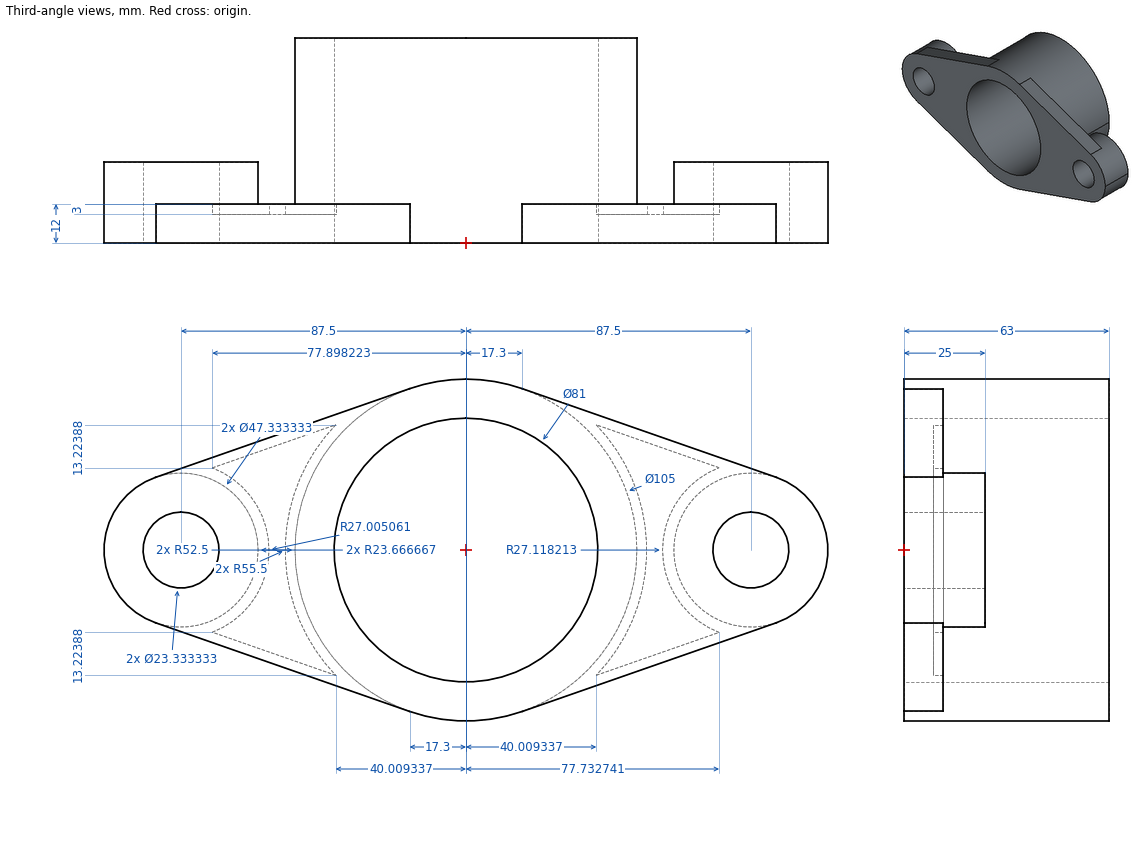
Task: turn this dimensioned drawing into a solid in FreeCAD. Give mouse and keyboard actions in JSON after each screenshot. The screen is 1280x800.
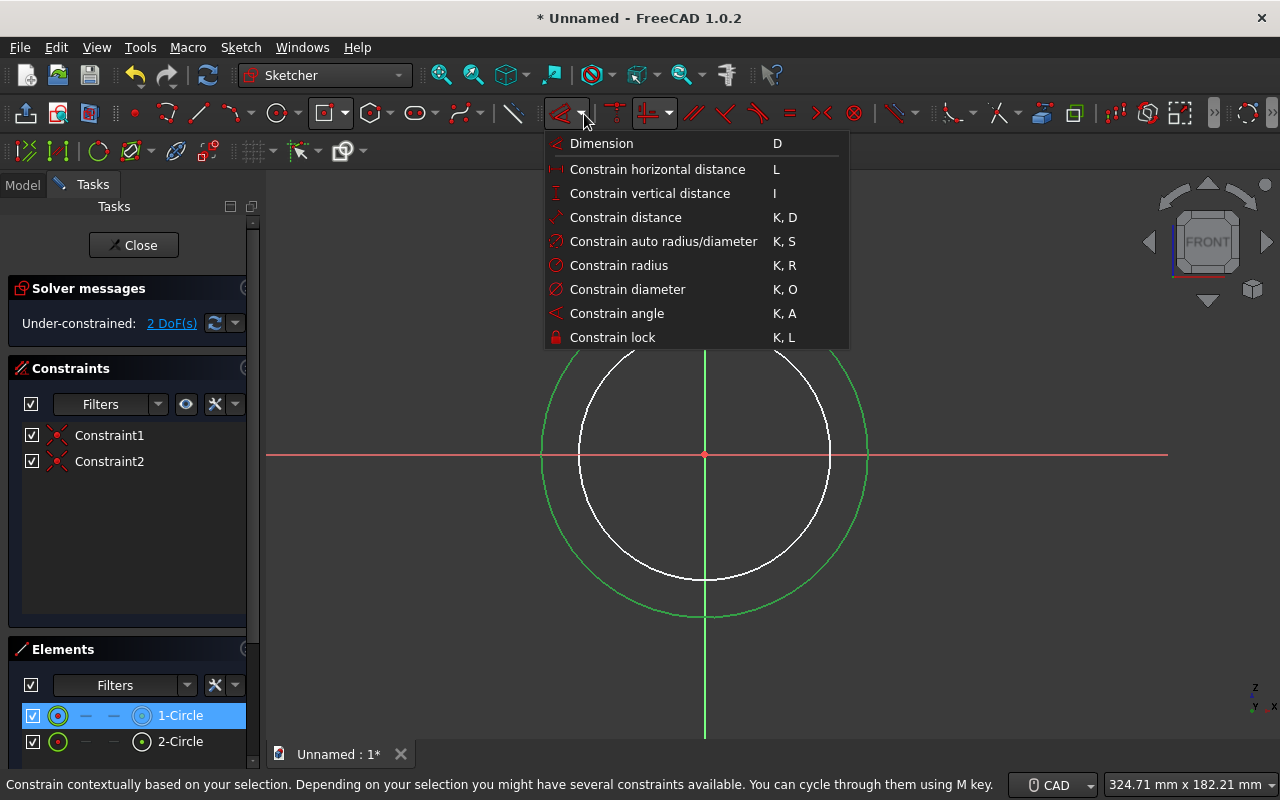
{"action": "left_click", "coordinate": [697, 289]}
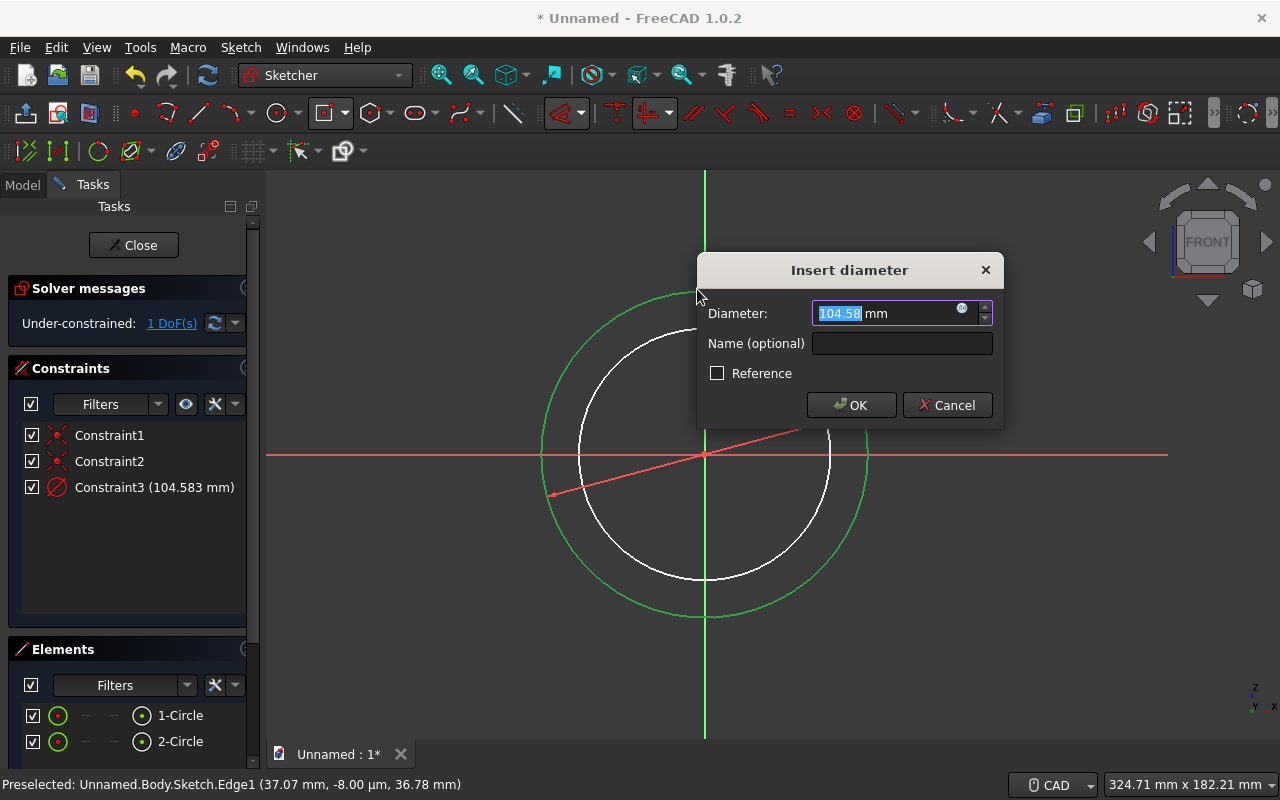
{"action": "type", "text": "105"}
{"action": "key", "text": "Return"}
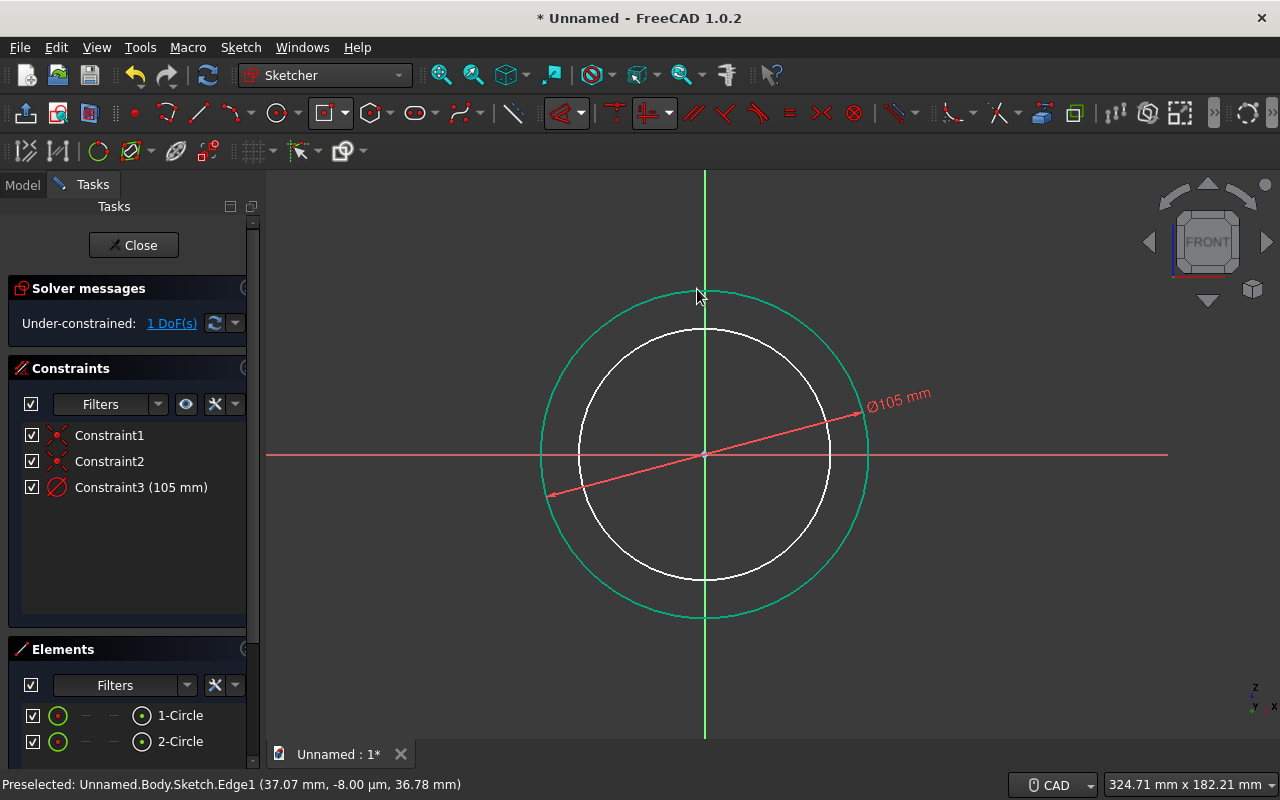
{"action": "left_click", "coordinate": [793, 365]}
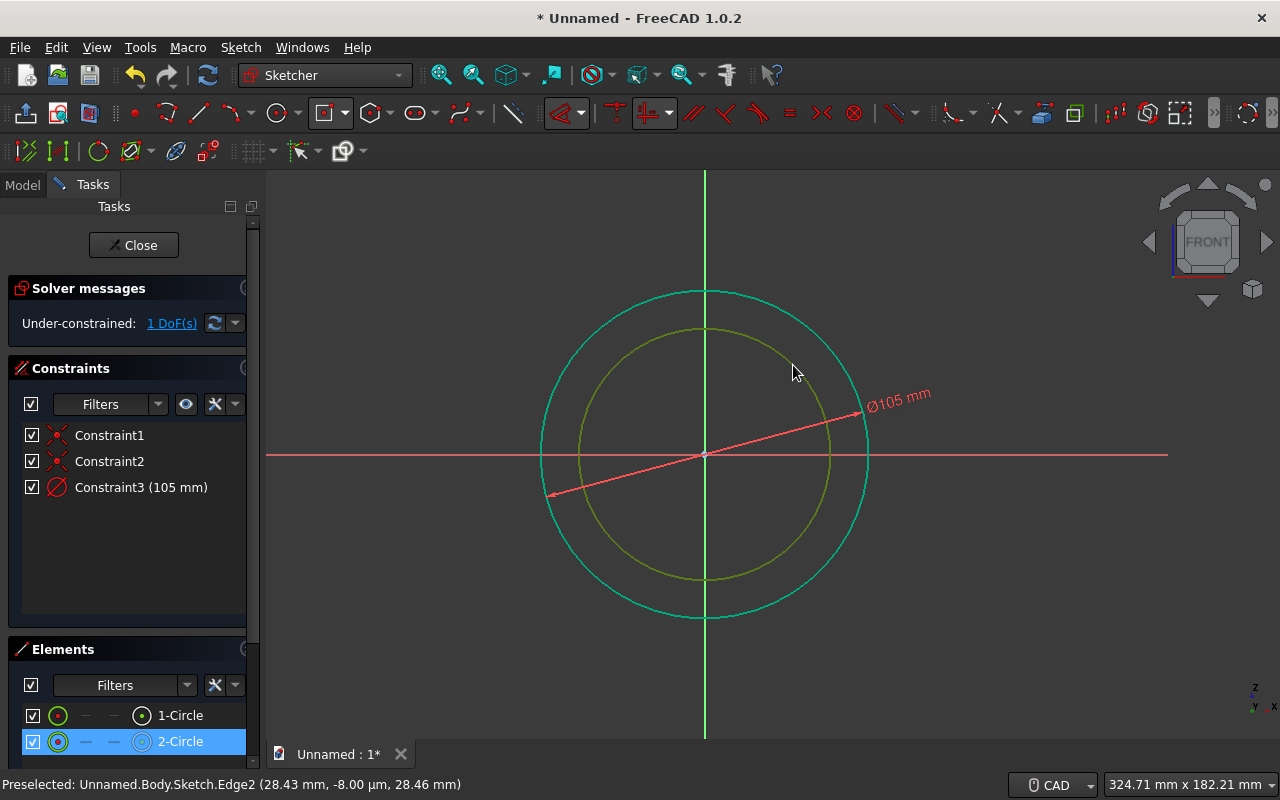
{"action": "key", "text": "k o"}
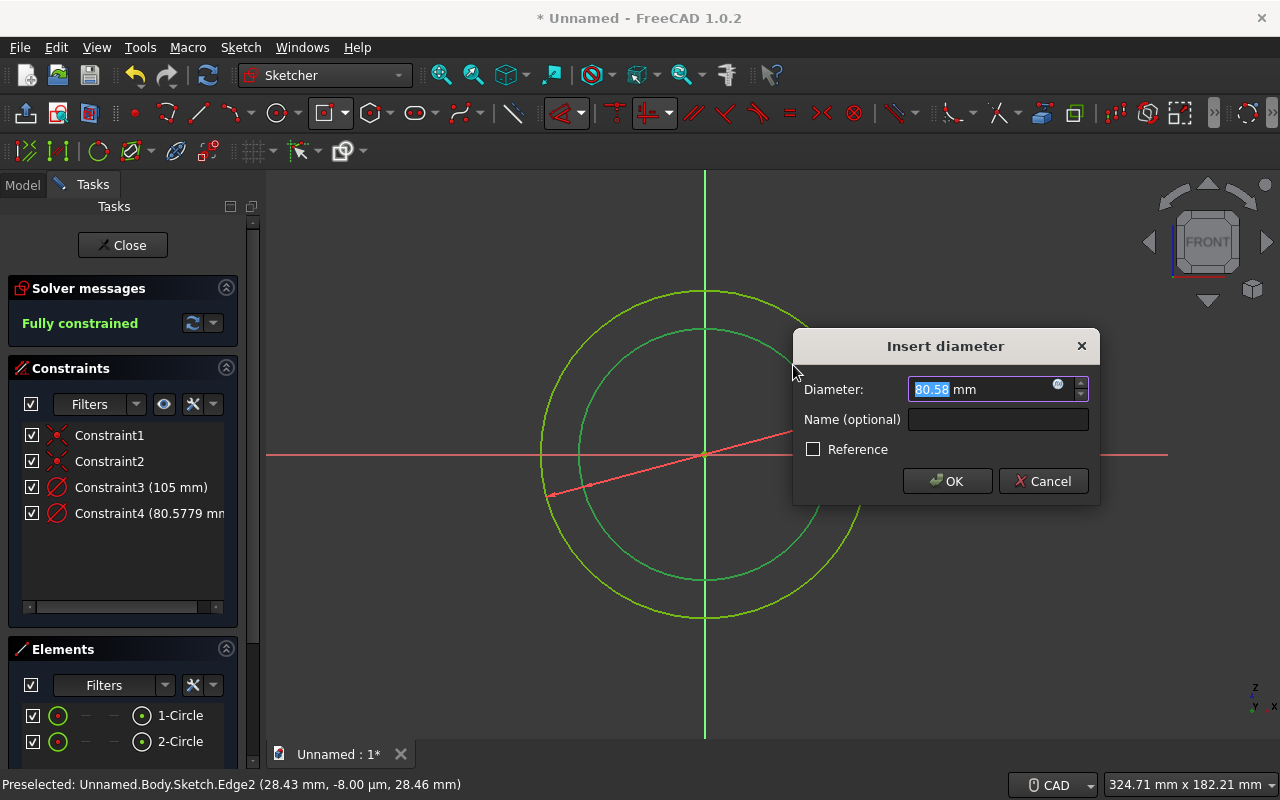
{"action": "type", "text": "81"}
{"action": "key", "text": "Return"}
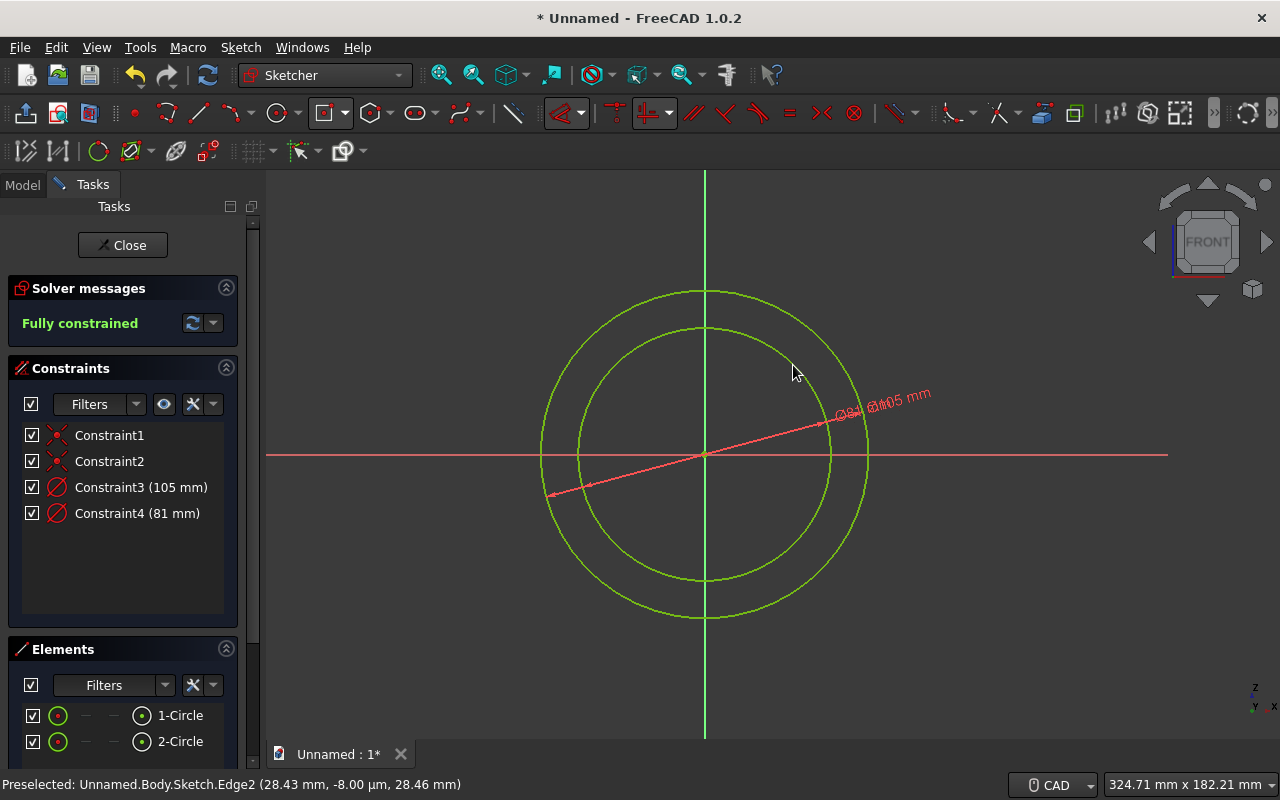
{"action": "left_click", "coordinate": [123, 245]}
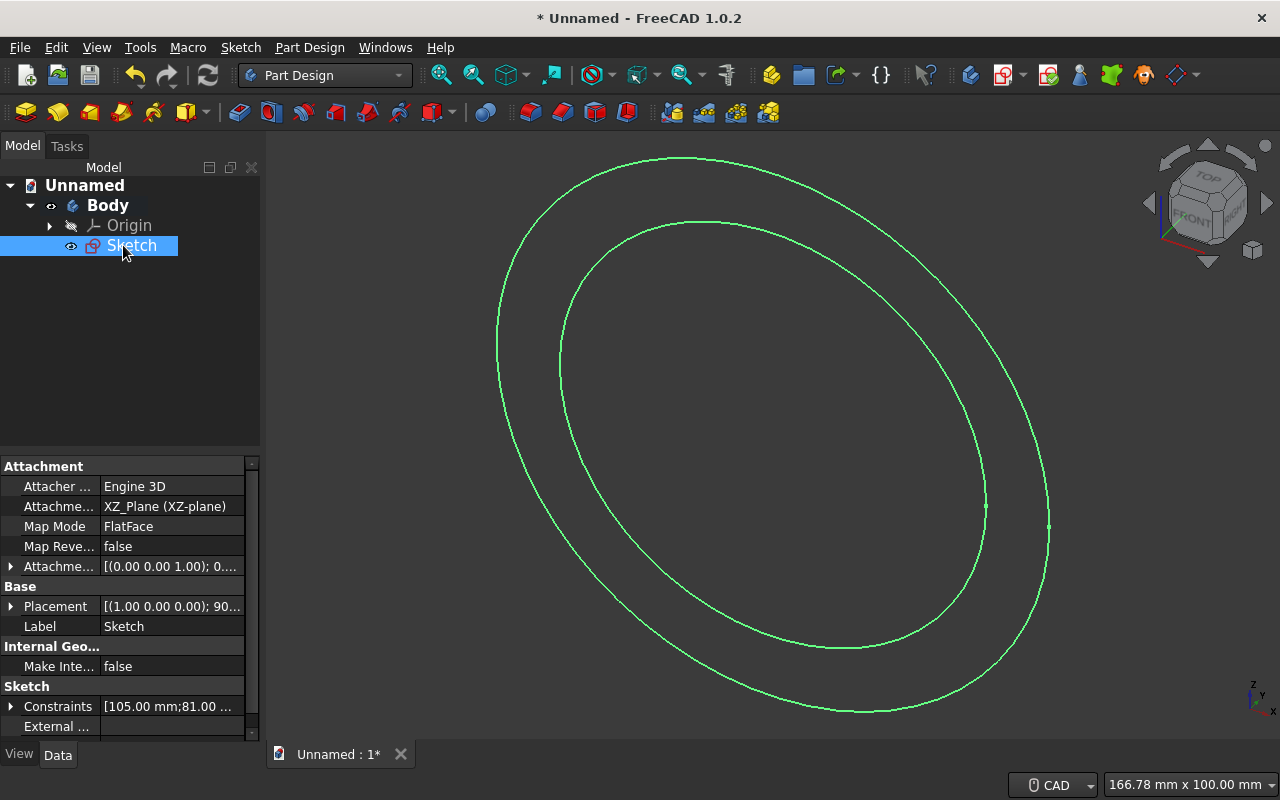
{"action": "left_click", "coordinate": [26, 112]}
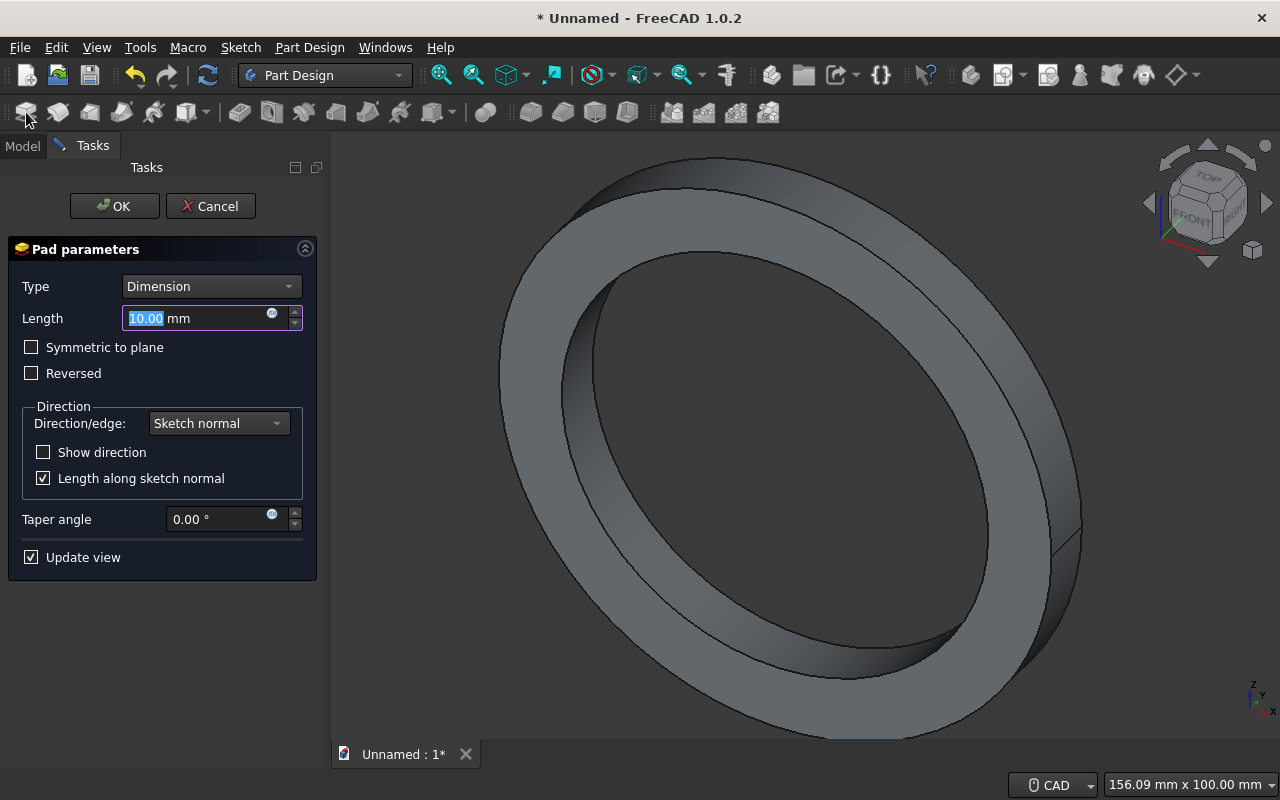
{"action": "type", "text": "63"}
{"action": "key", "text": "Tab"}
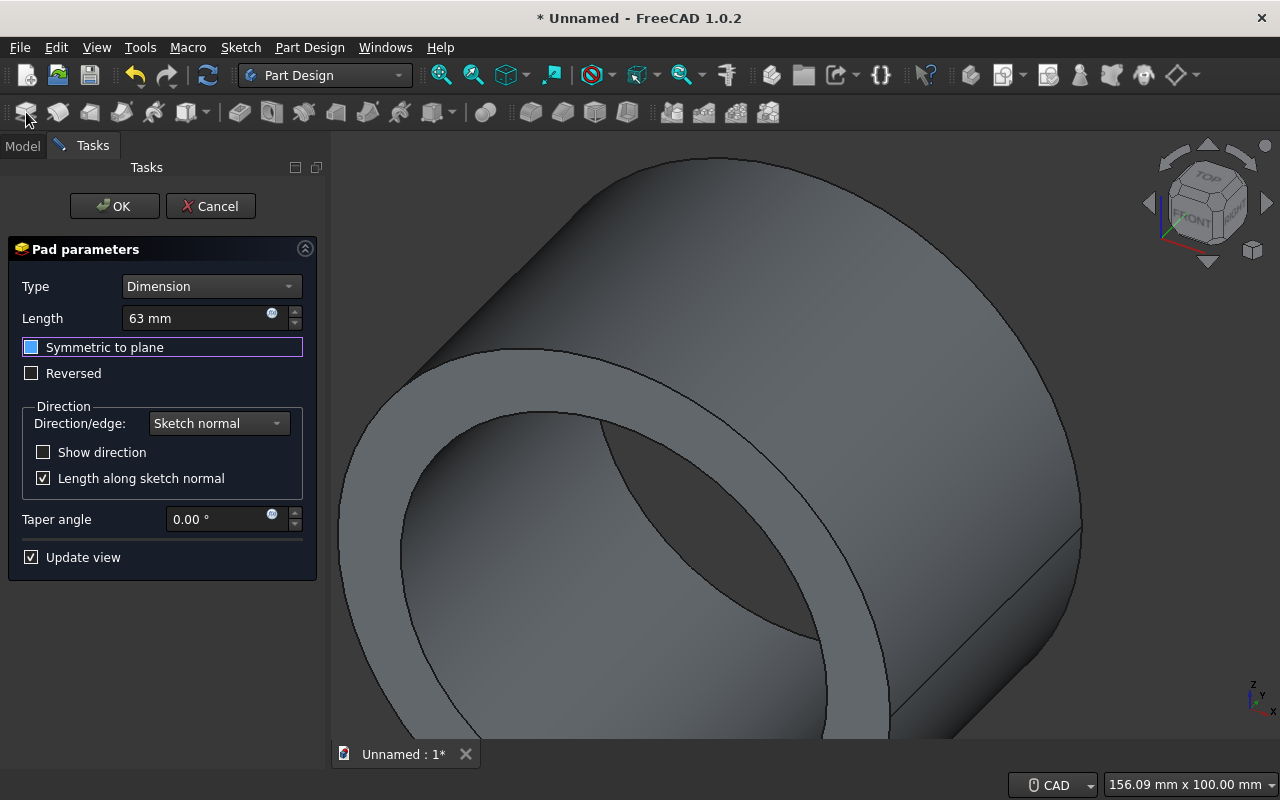
{"action": "left_click", "coordinate": [30, 373]}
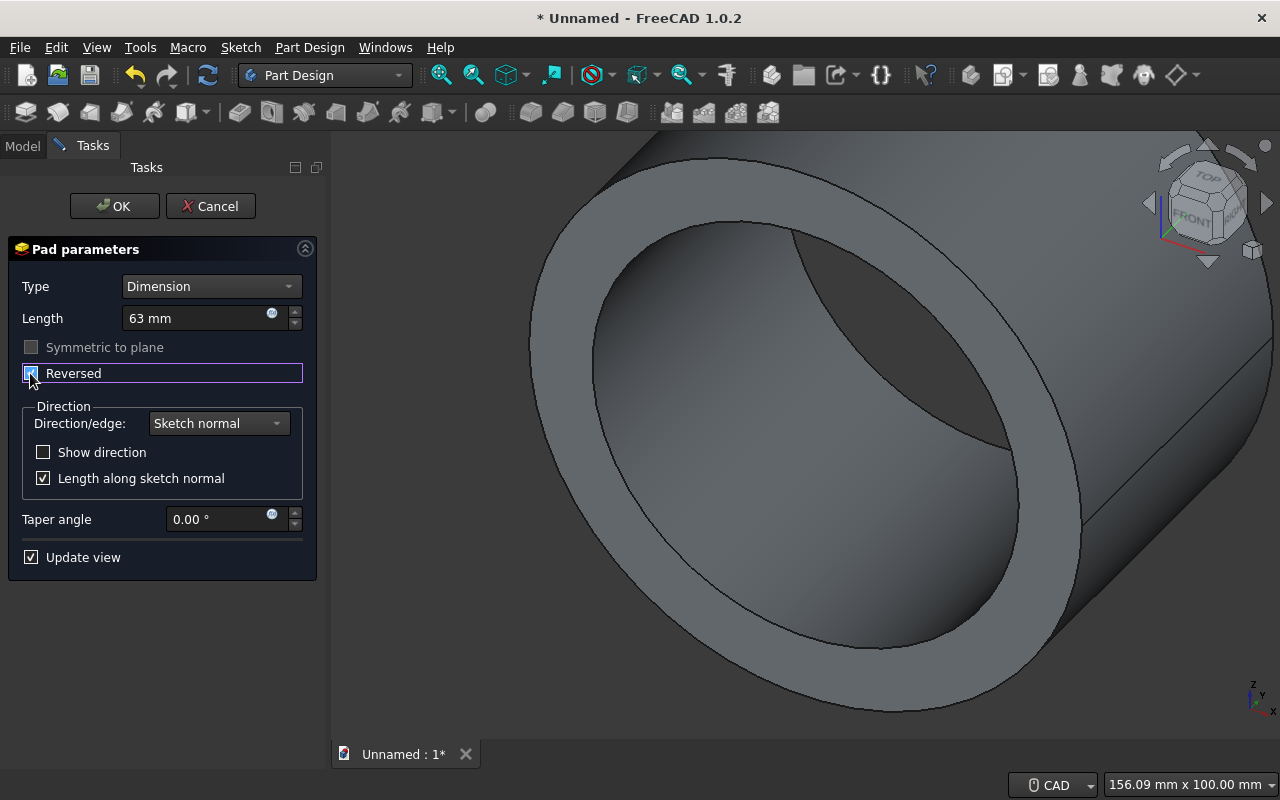
{"action": "left_click", "coordinate": [115, 206]}